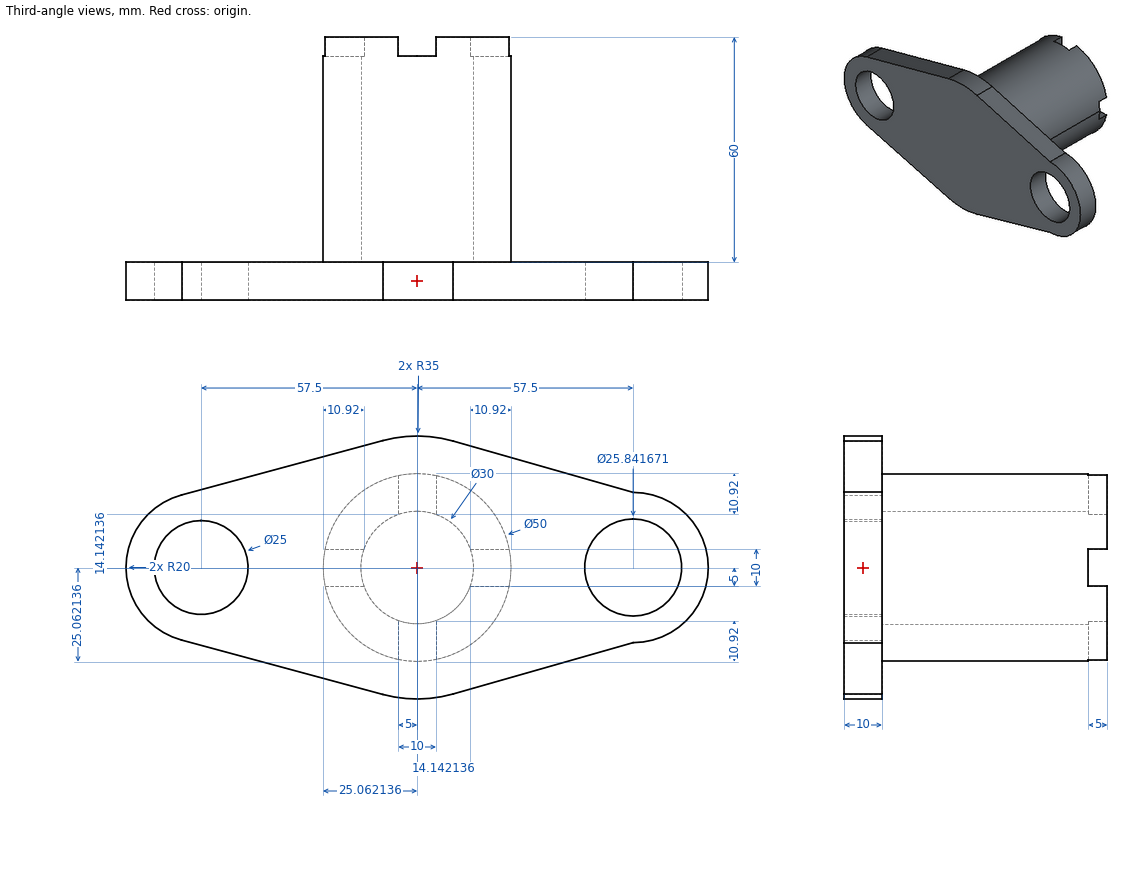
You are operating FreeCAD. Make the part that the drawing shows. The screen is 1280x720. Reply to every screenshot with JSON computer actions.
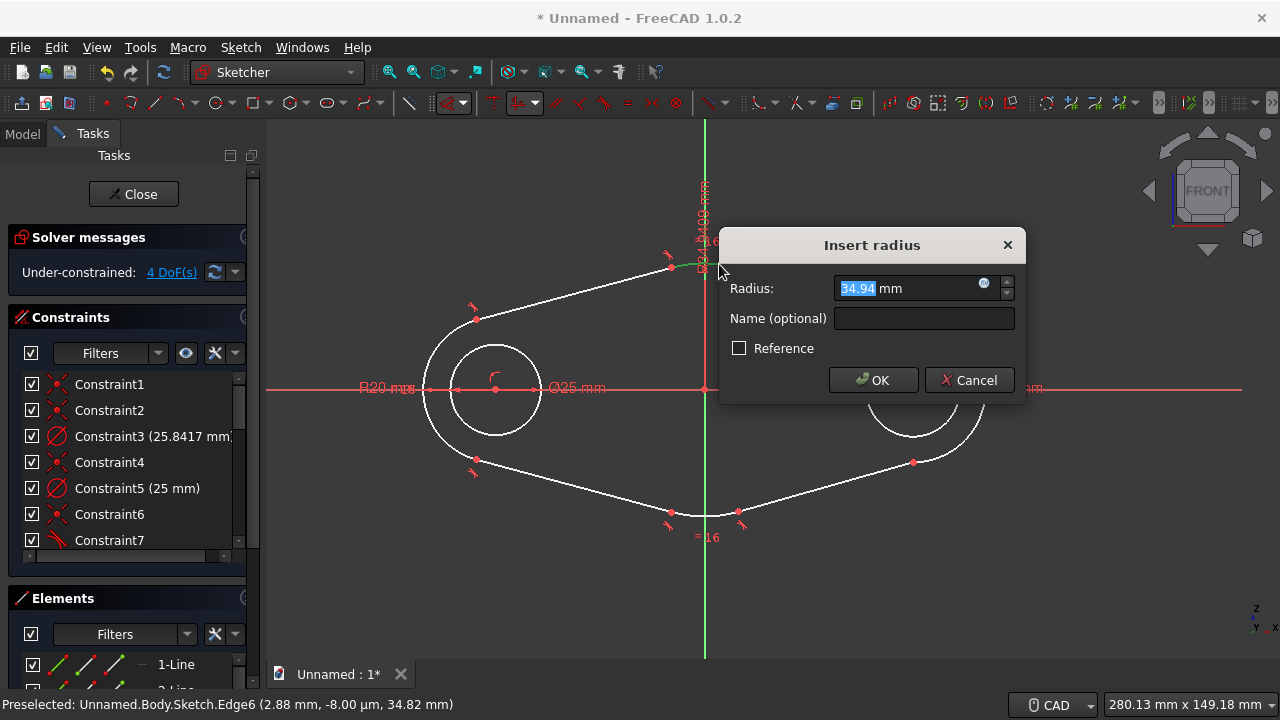
{"action": "type", "text": "35"}
{"action": "key", "text": "Return"}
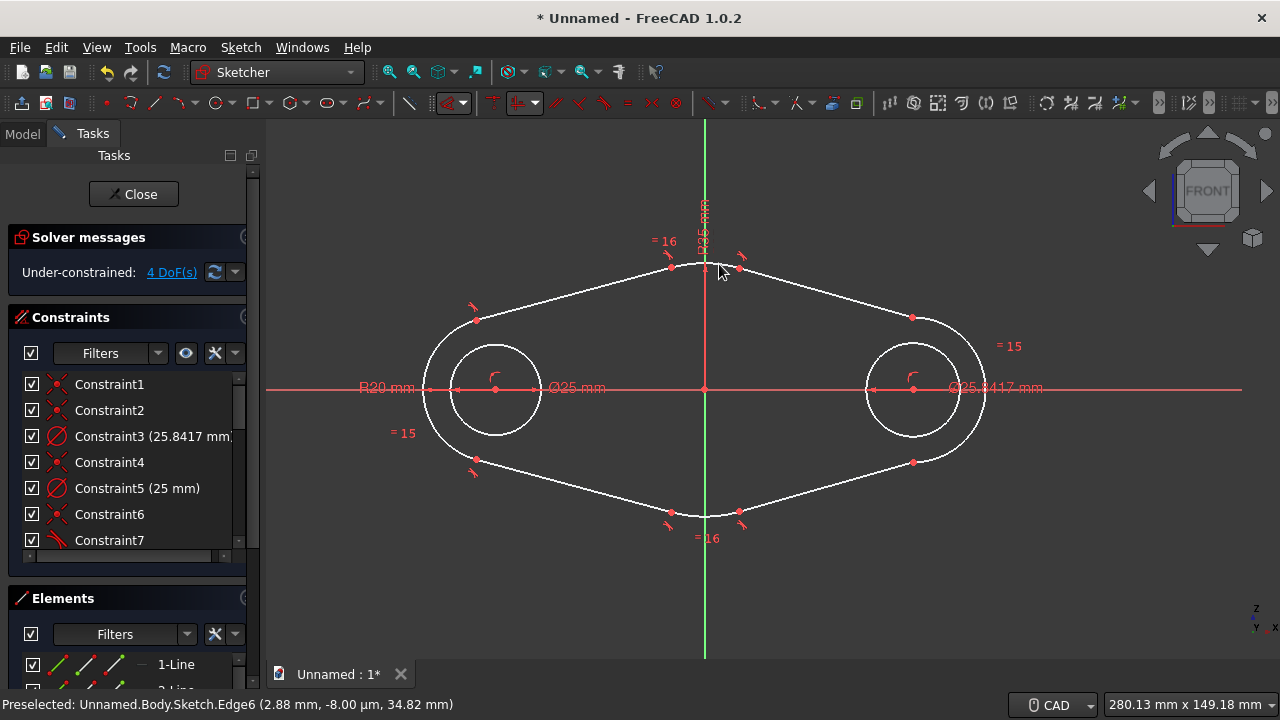
{"action": "left_click", "coordinate": [913, 390]}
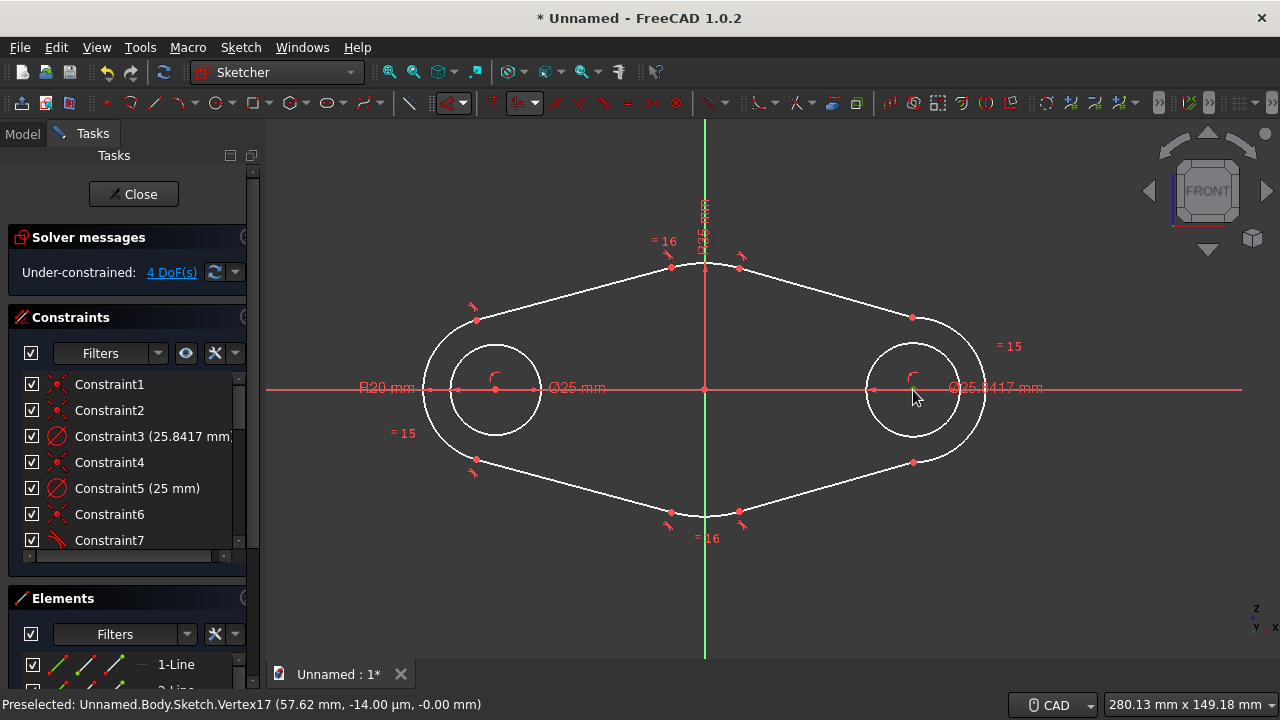
{"action": "key", "text": "l"}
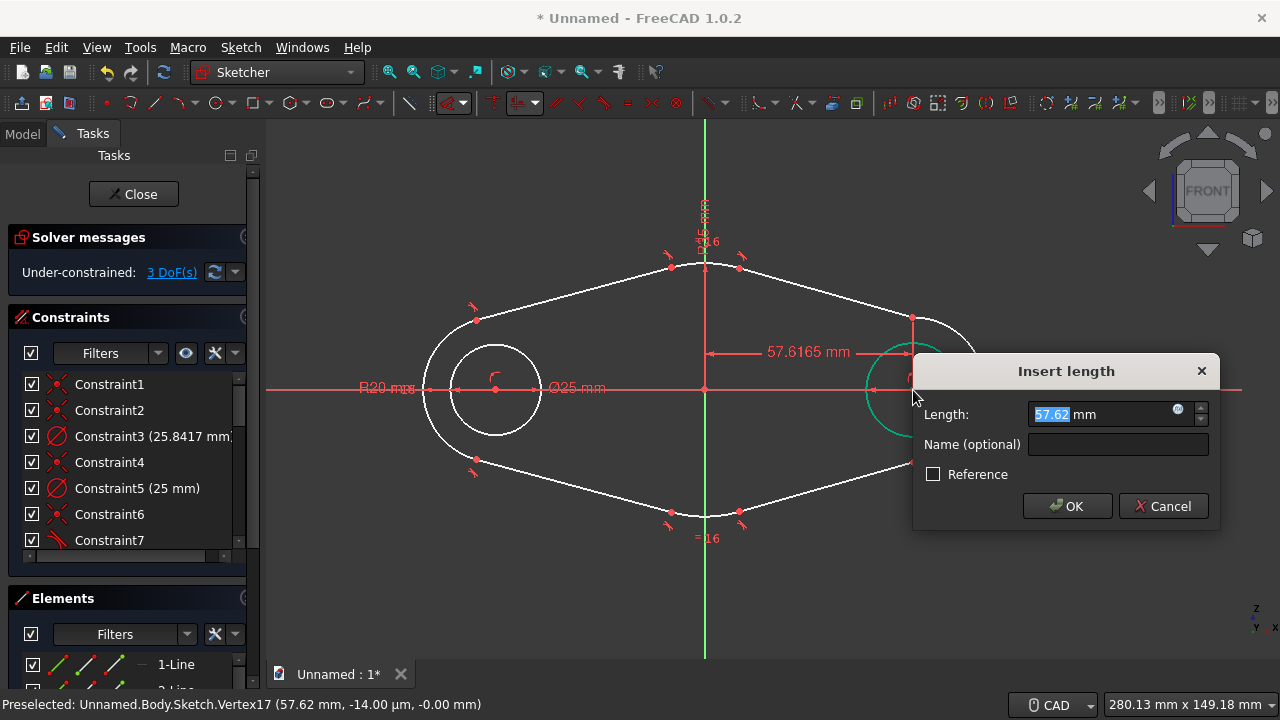
{"action": "type", "text": "57.5"}
{"action": "key", "text": "Return"}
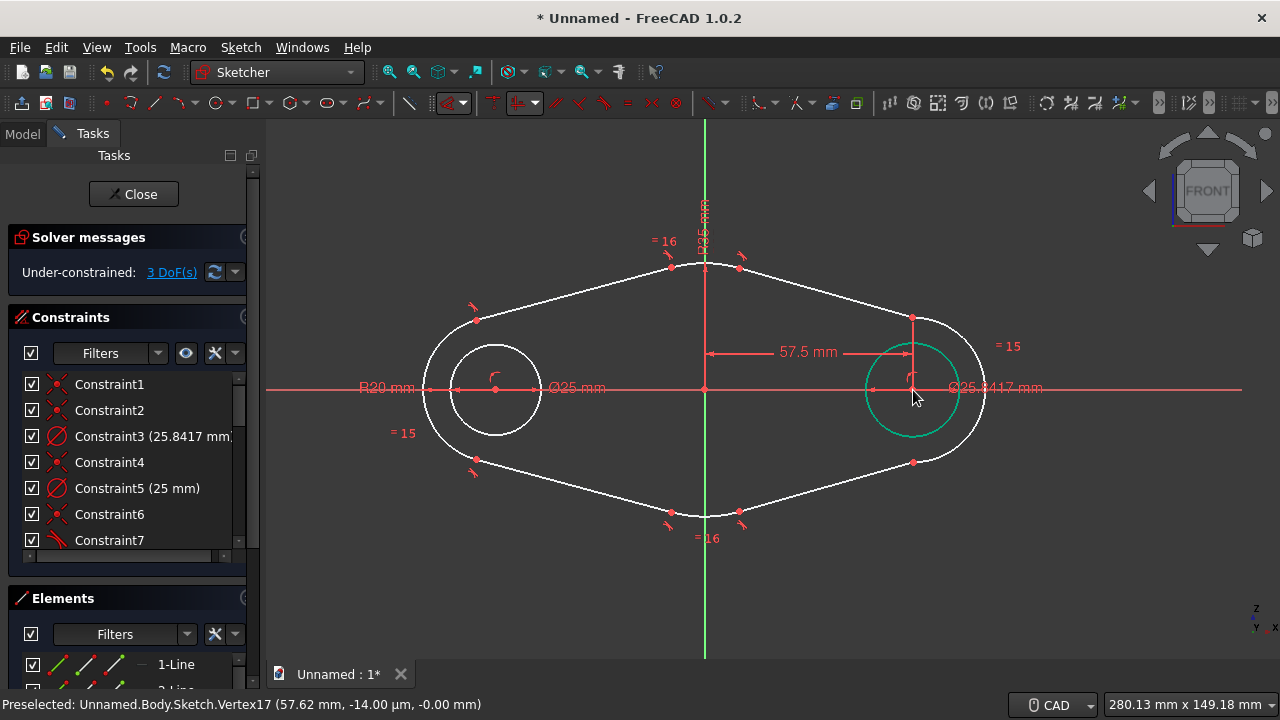
{"action": "left_click", "coordinate": [496, 390]}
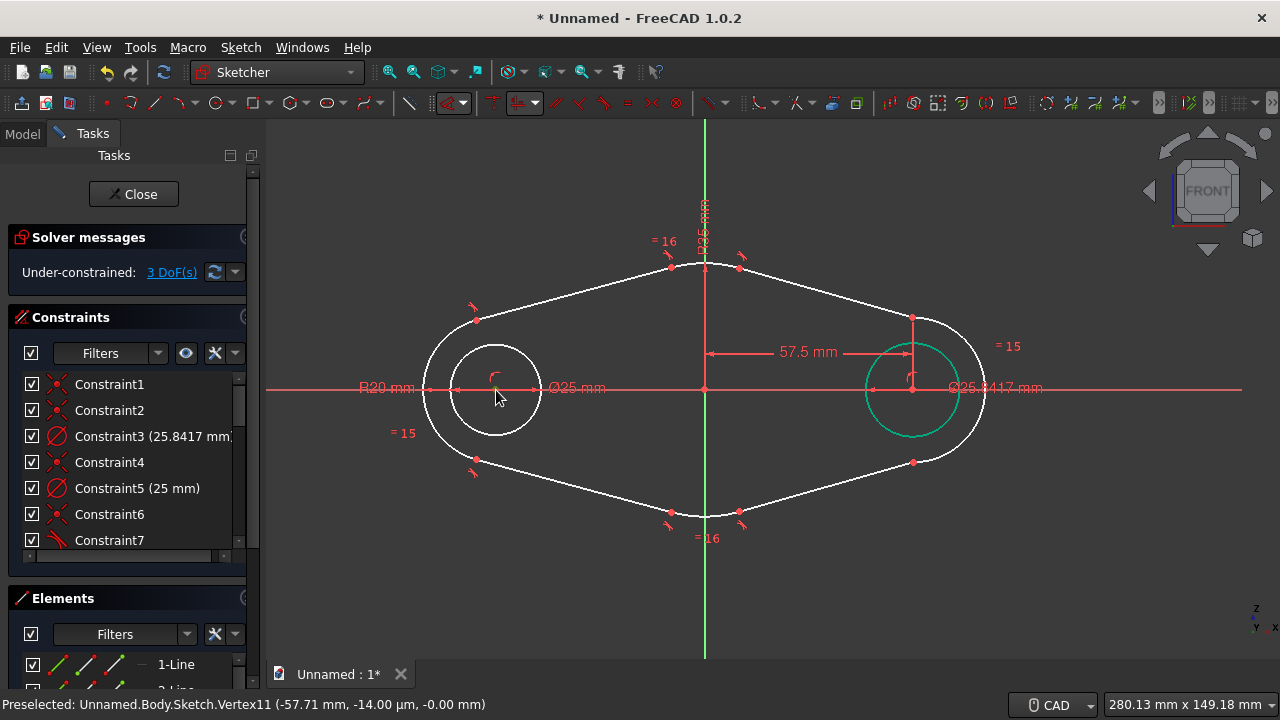
{"action": "key", "text": "l"}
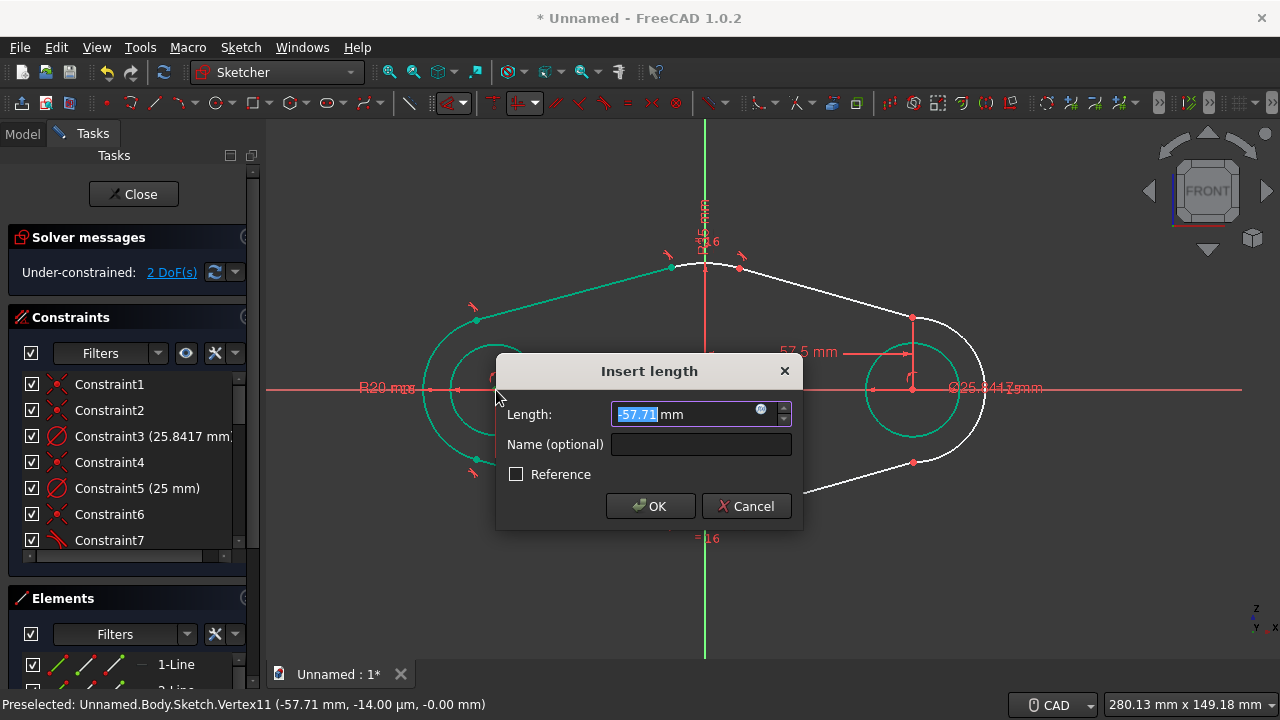
{"action": "type", "text": "-57.5"}
{"action": "key", "text": "Return"}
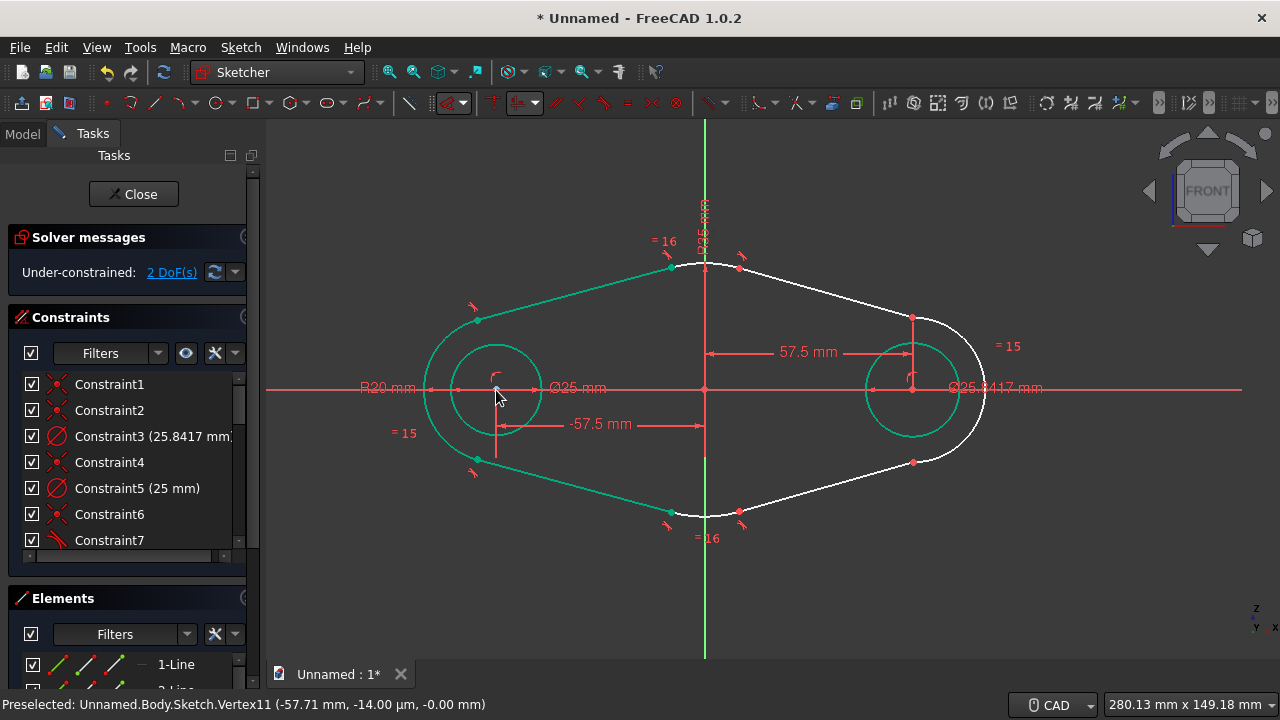
{"action": "left_click", "coordinate": [913, 318]}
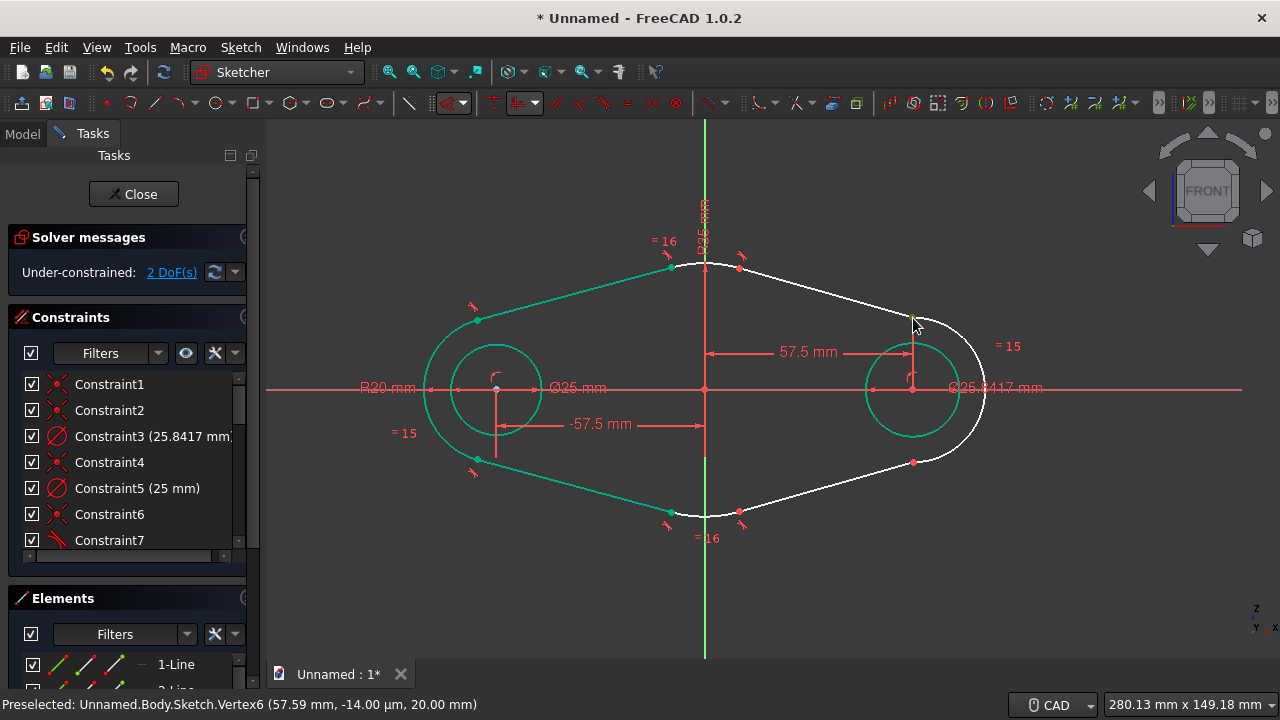
{"action": "key", "text": "l"}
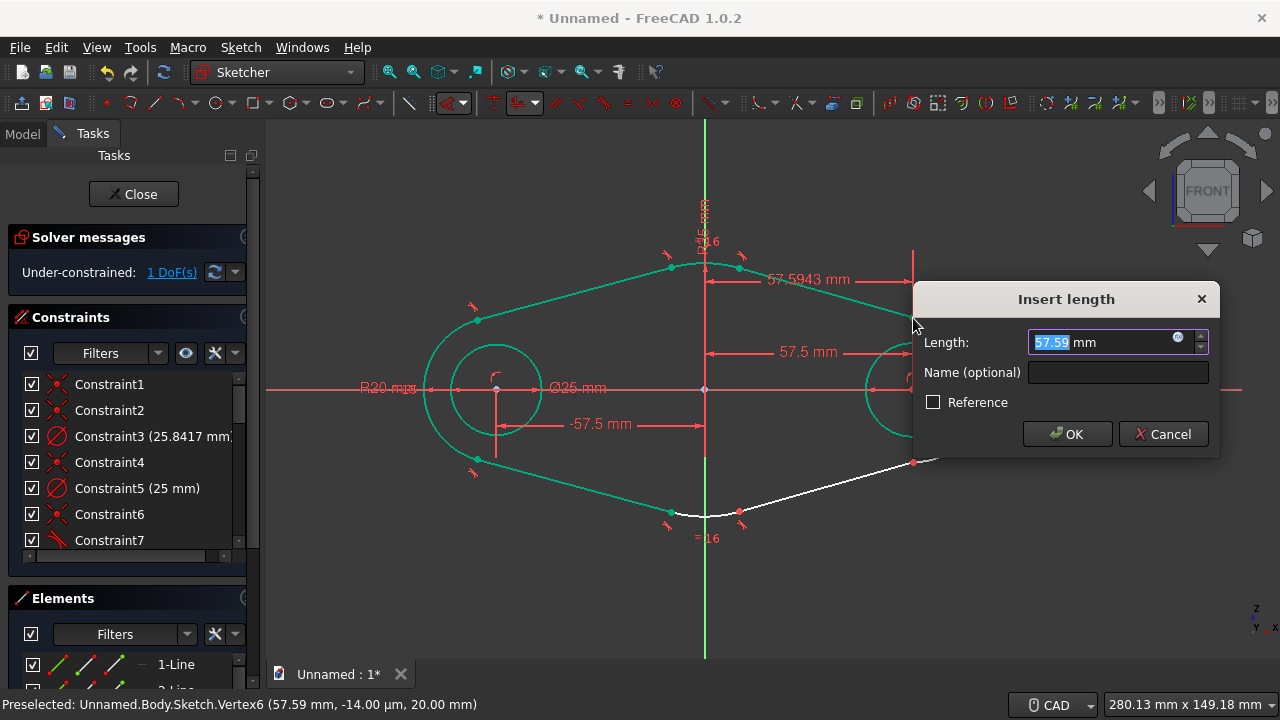
{"action": "type", "text": "57.5"}
{"action": "key", "text": "Return"}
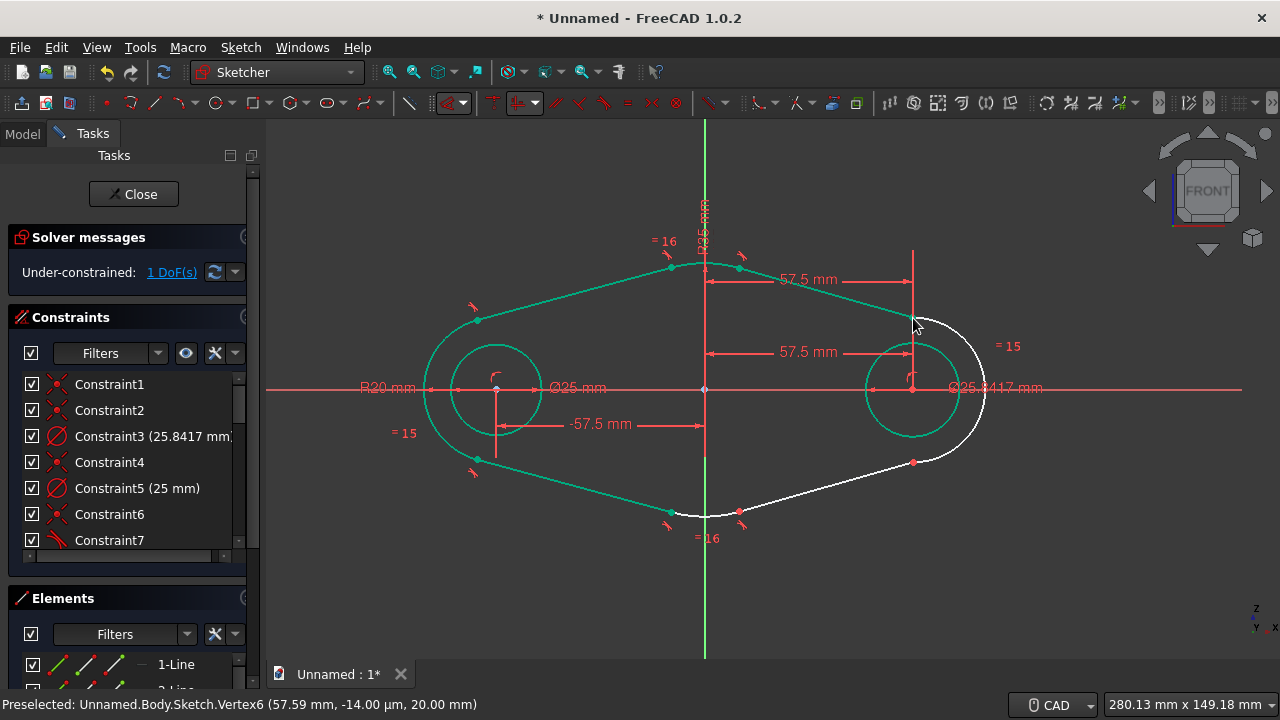
{"action": "left_click", "coordinate": [913, 462]}